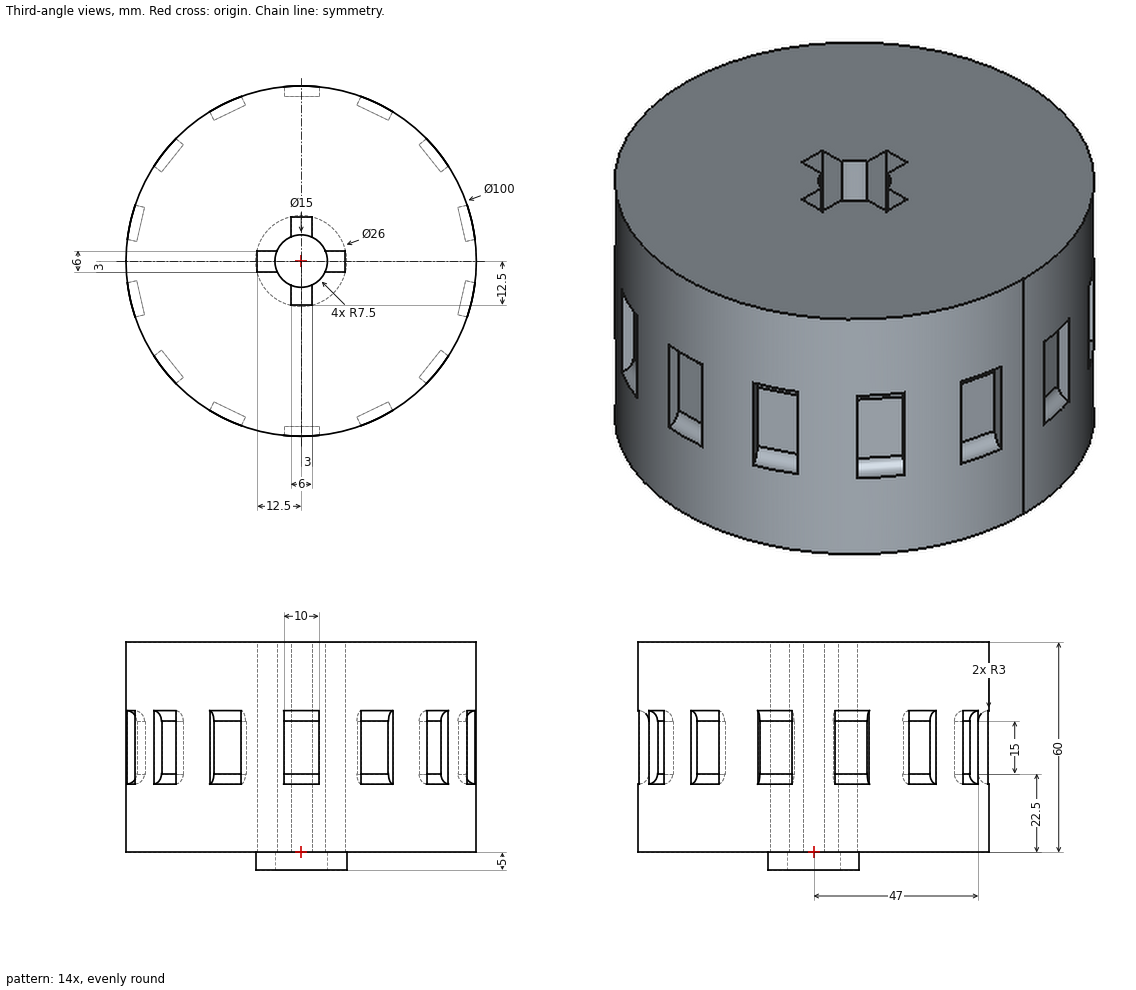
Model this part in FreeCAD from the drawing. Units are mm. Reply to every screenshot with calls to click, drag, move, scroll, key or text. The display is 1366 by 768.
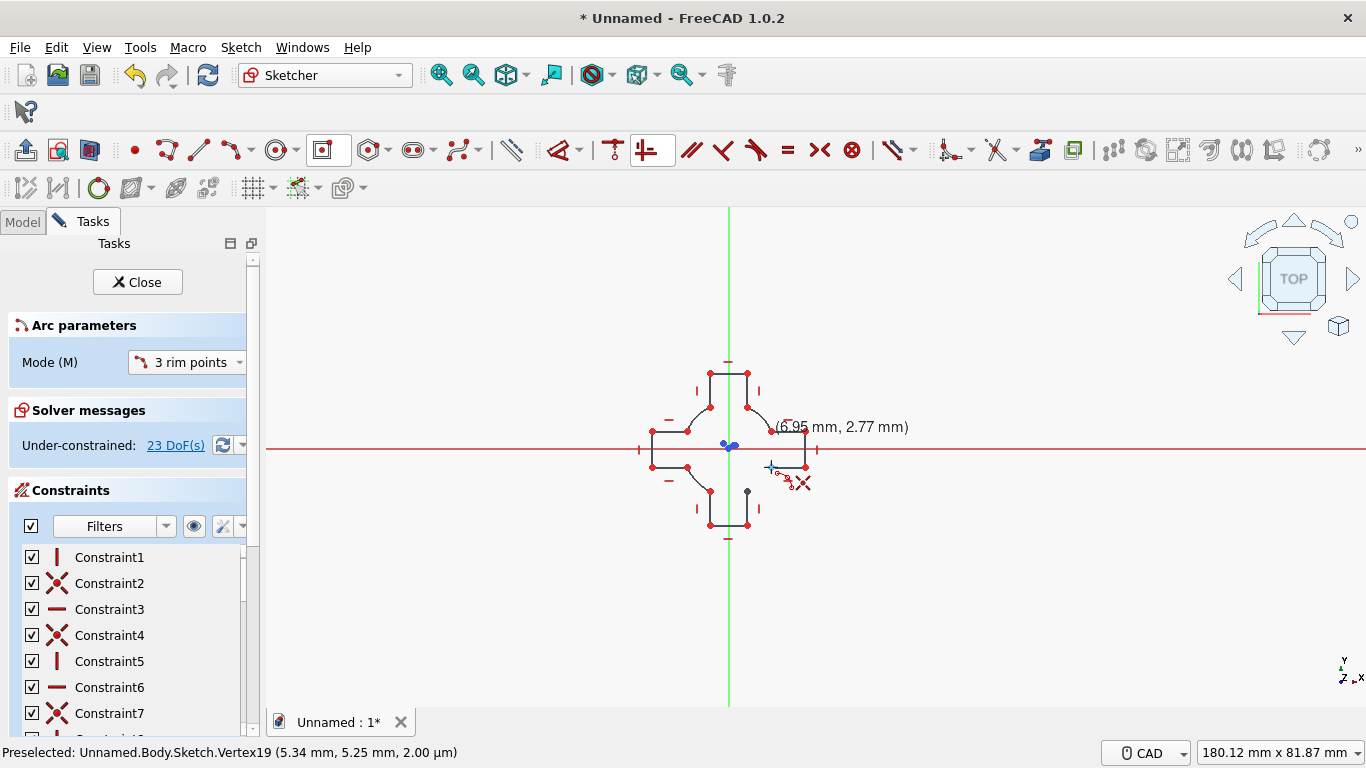
click(771, 468)
click(747, 492)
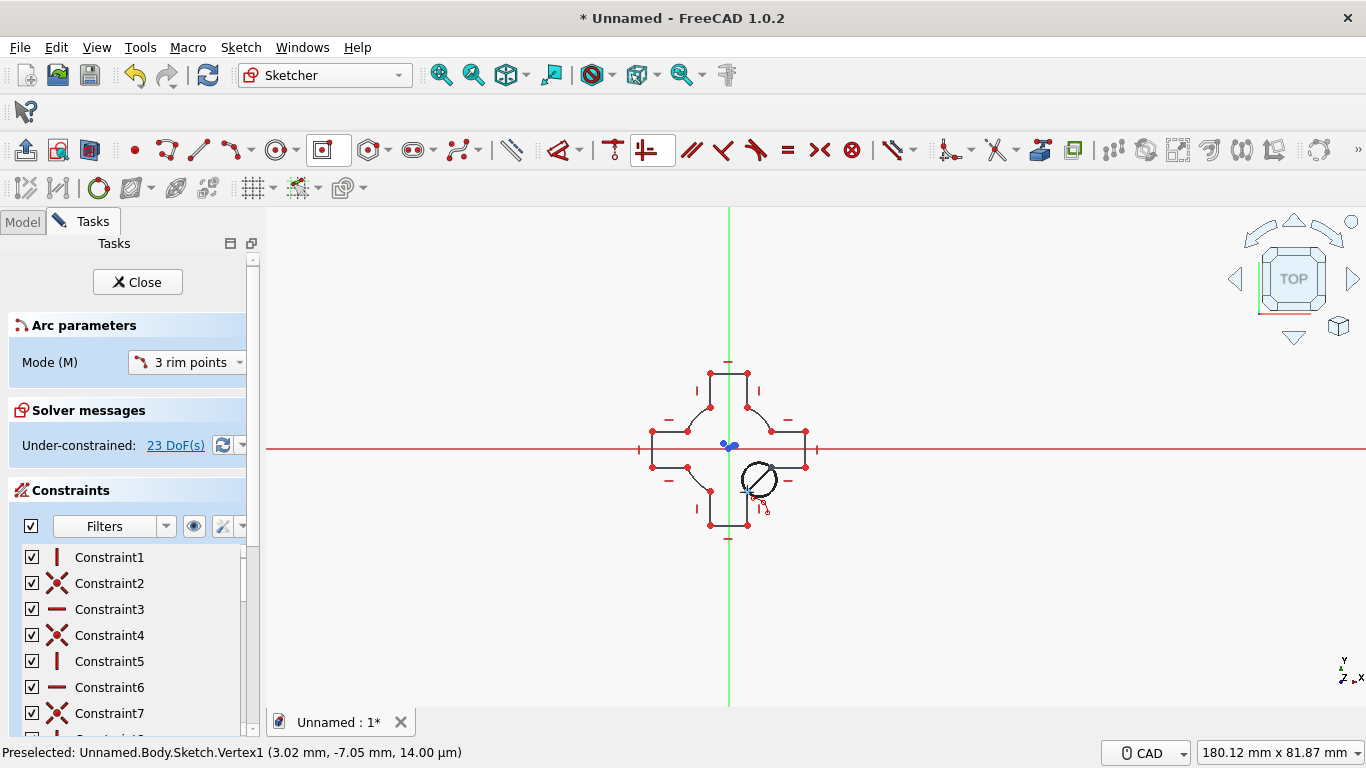
scroll(761, 481, up, 9)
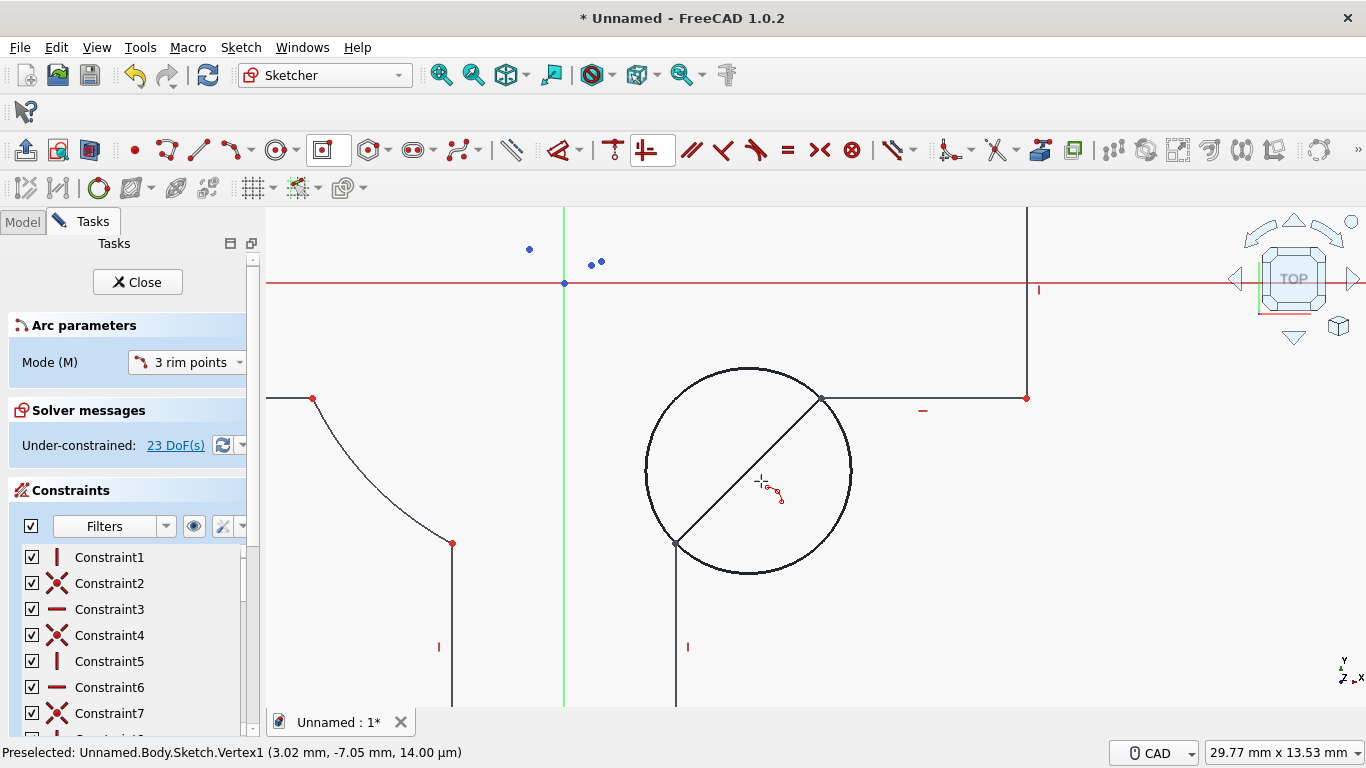
click(760, 479)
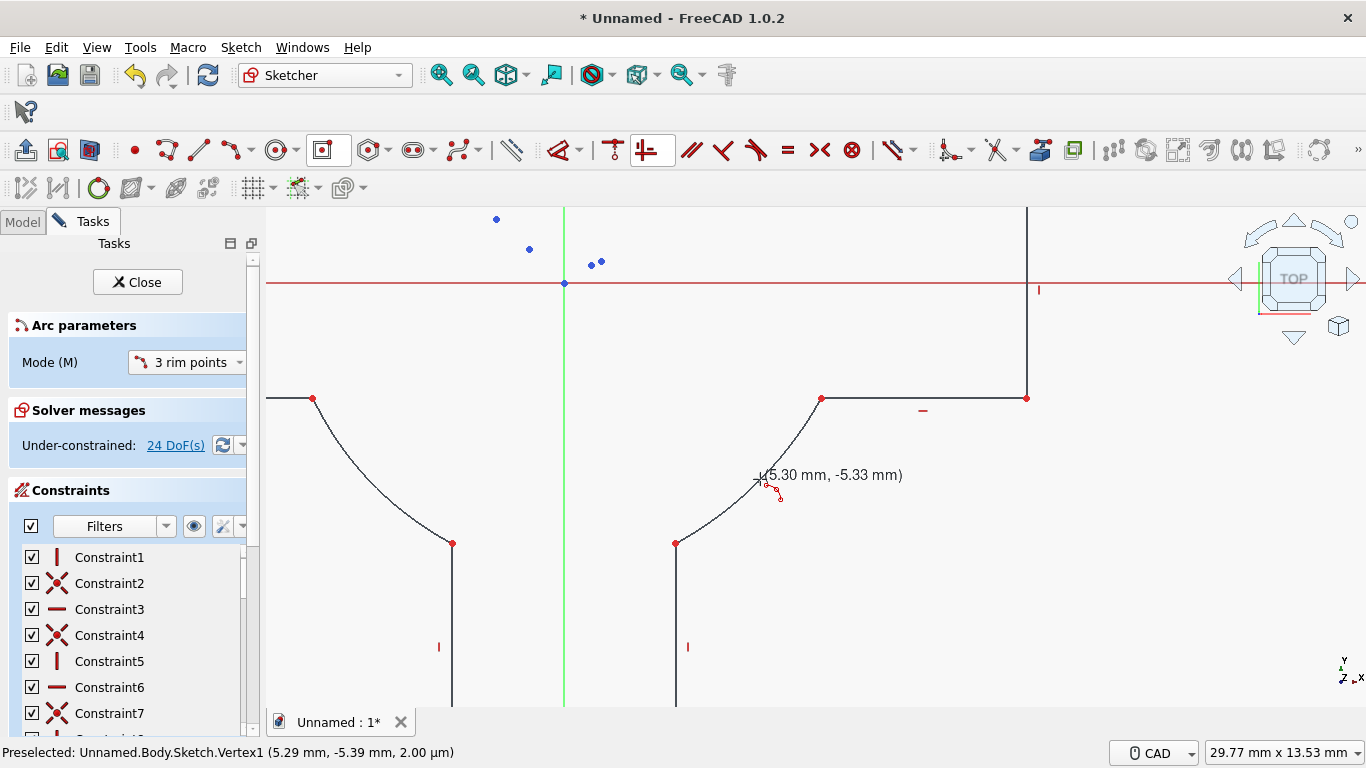
key(g)
key(c)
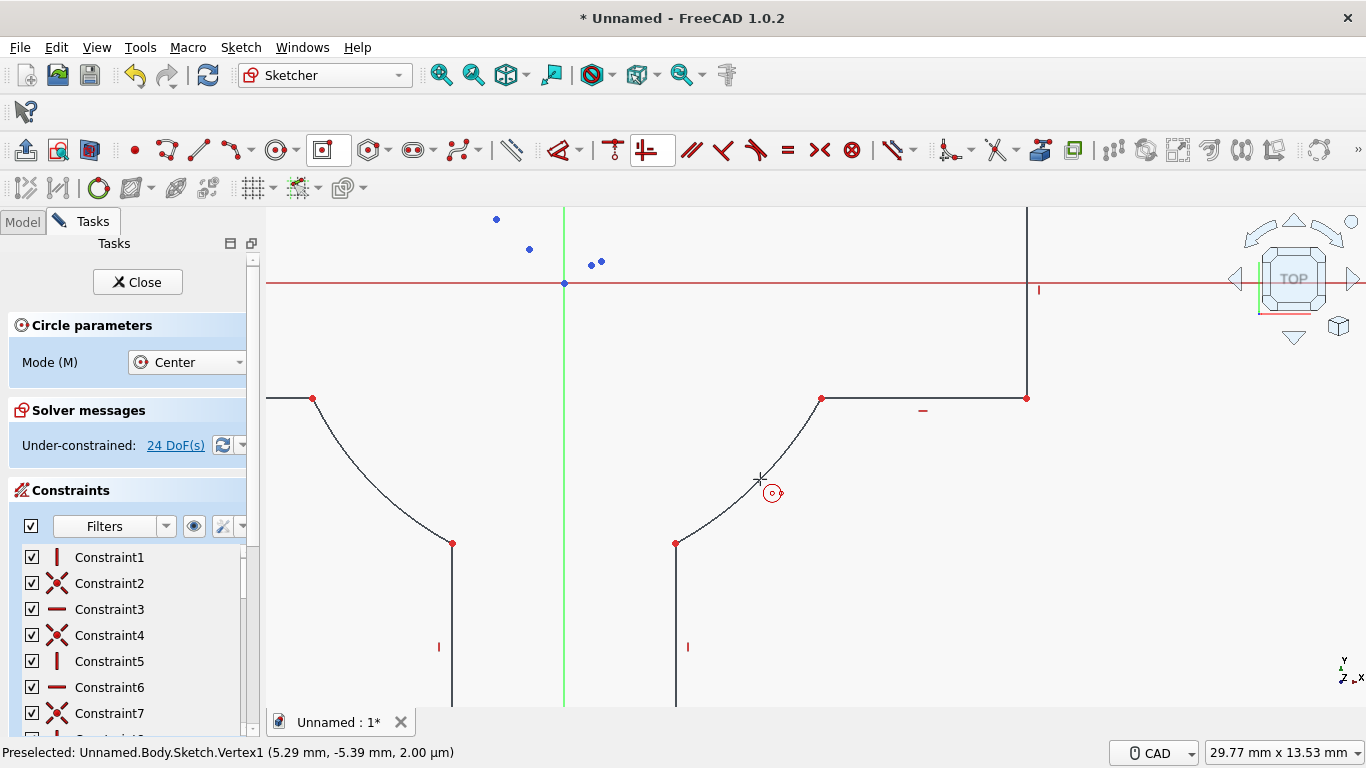
scroll(766, 474, down, 12)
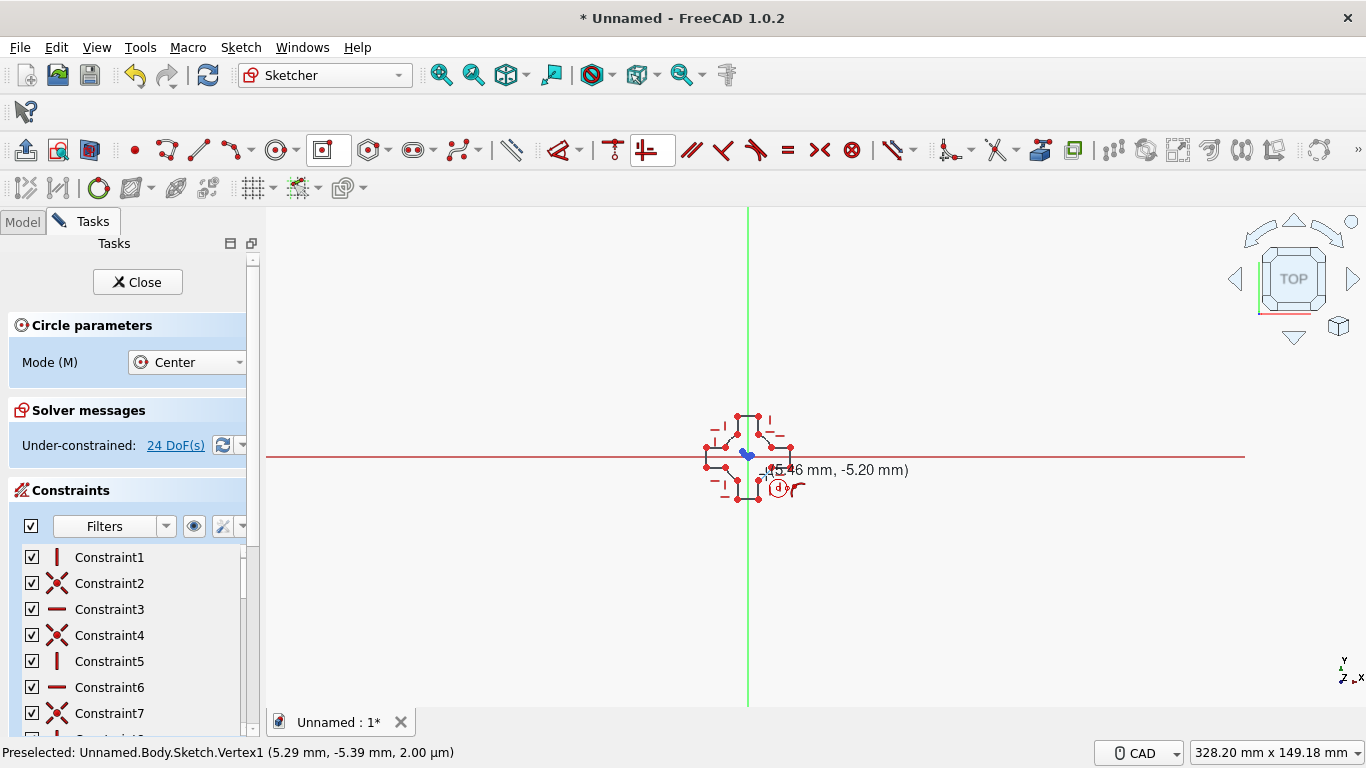
click(748, 457)
click(867, 339)
key(Escape)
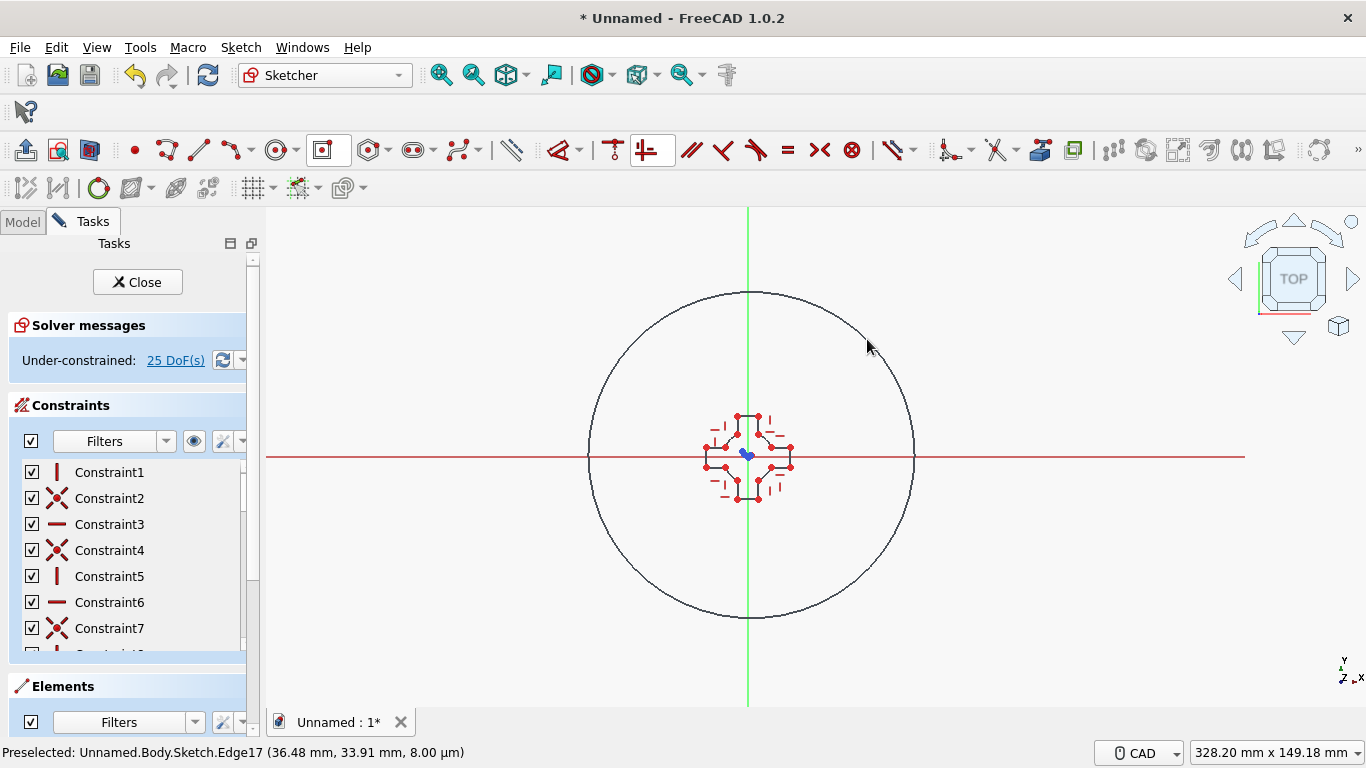
click(866, 339)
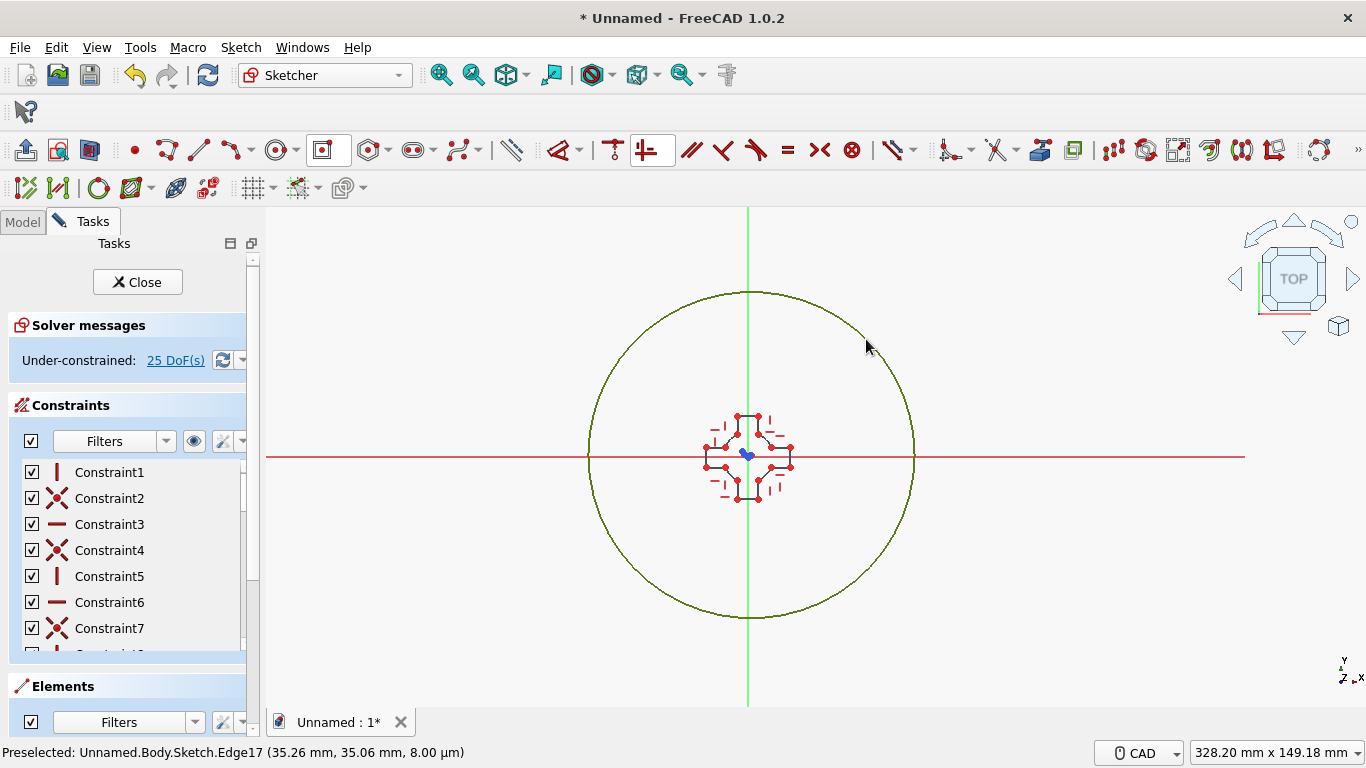
scroll(730, 440, up, 2)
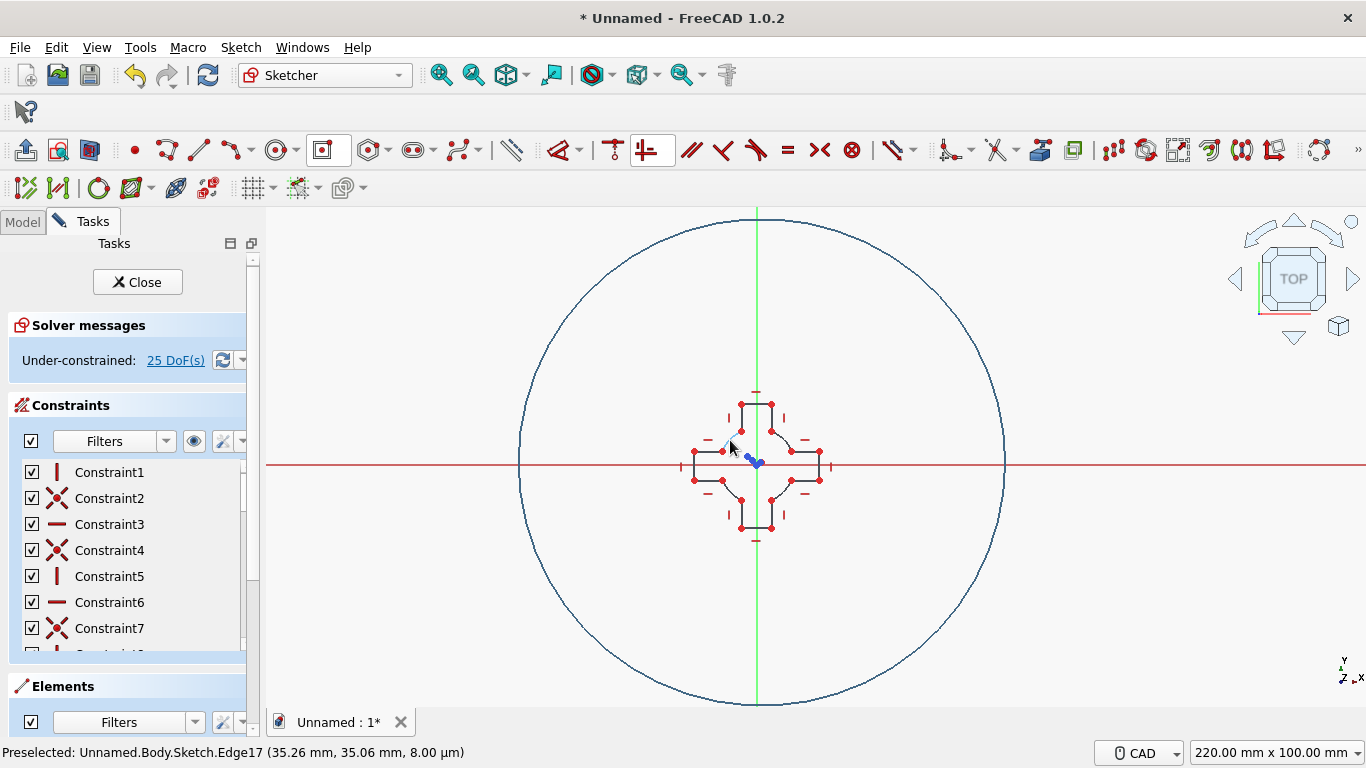
click(730, 439)